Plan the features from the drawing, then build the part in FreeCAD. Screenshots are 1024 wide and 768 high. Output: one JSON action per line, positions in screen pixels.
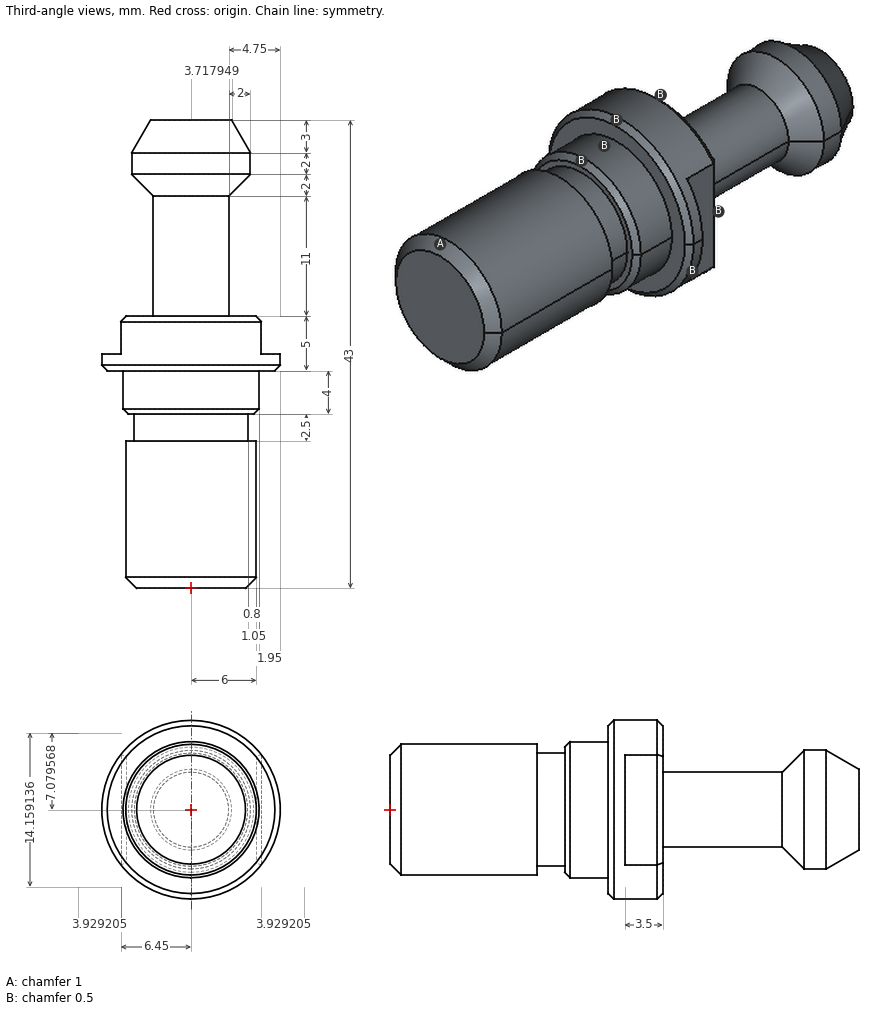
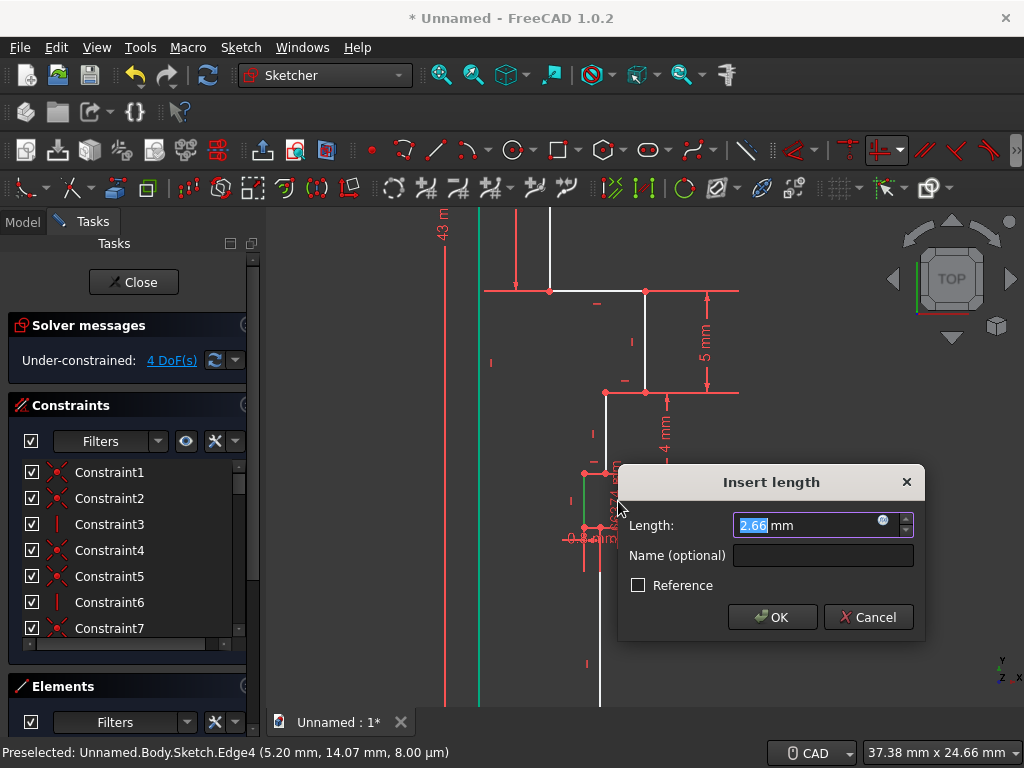
{"action": "type", "text": "2.5"}
{"action": "key", "text": "Return"}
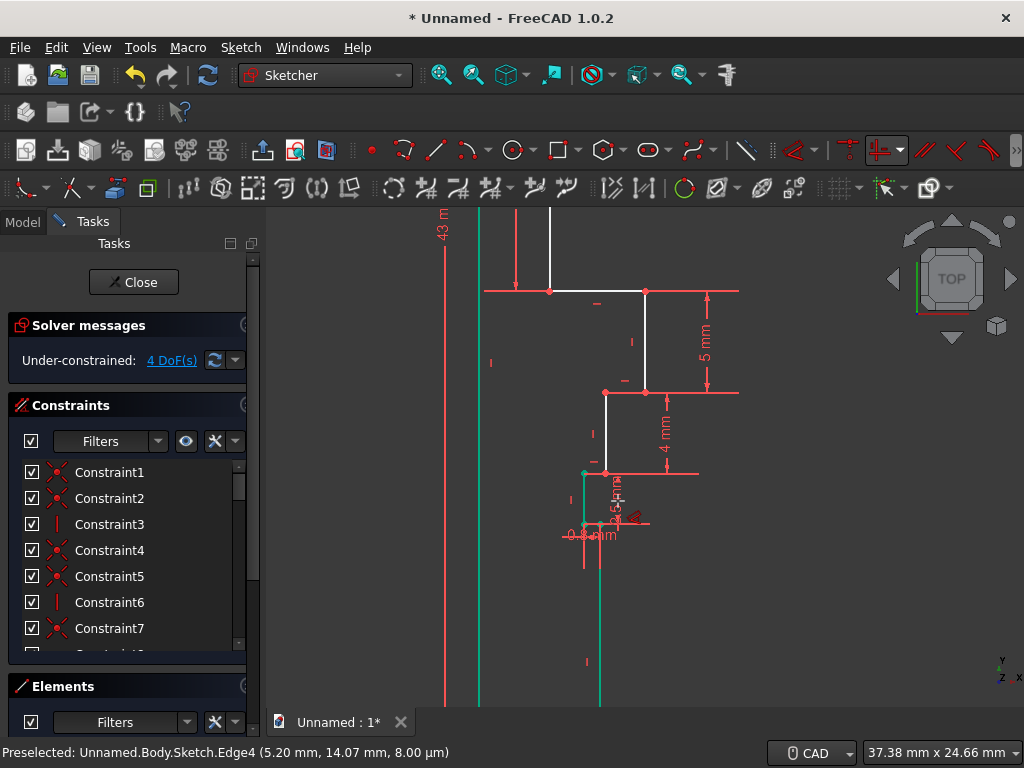
{"action": "scroll", "coordinate": [595, 474], "scroll_direction": "up", "scroll_amount": 4}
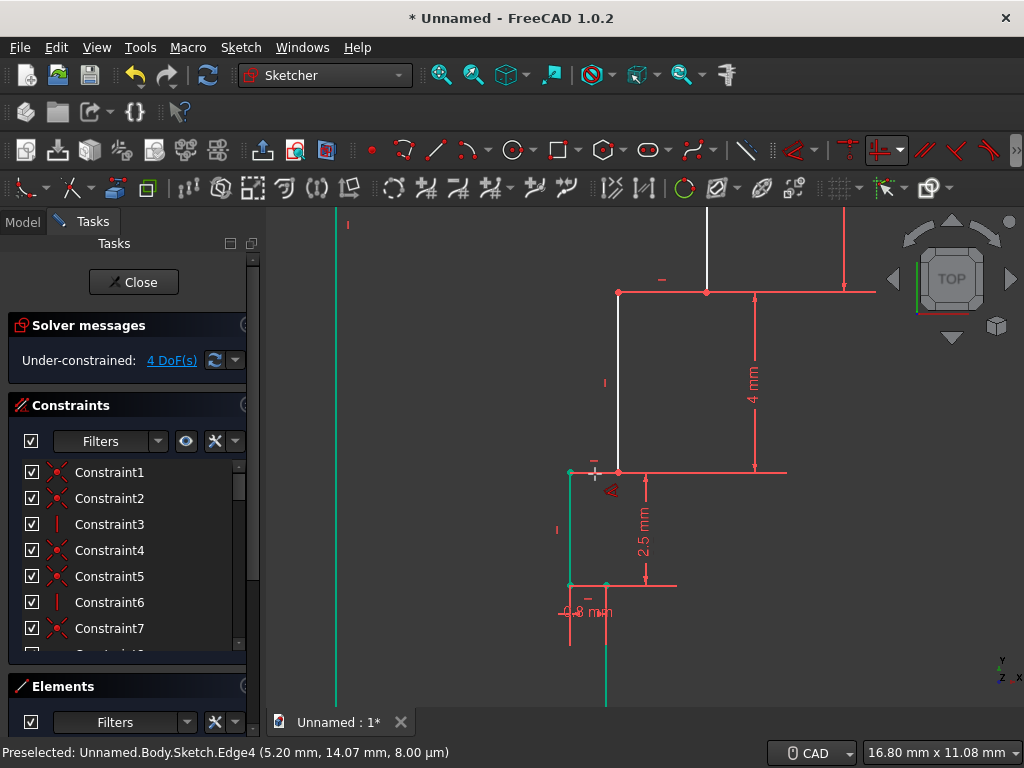
{"action": "left_click", "coordinate": [594, 473]}
{"action": "left_click", "coordinate": [594, 507]}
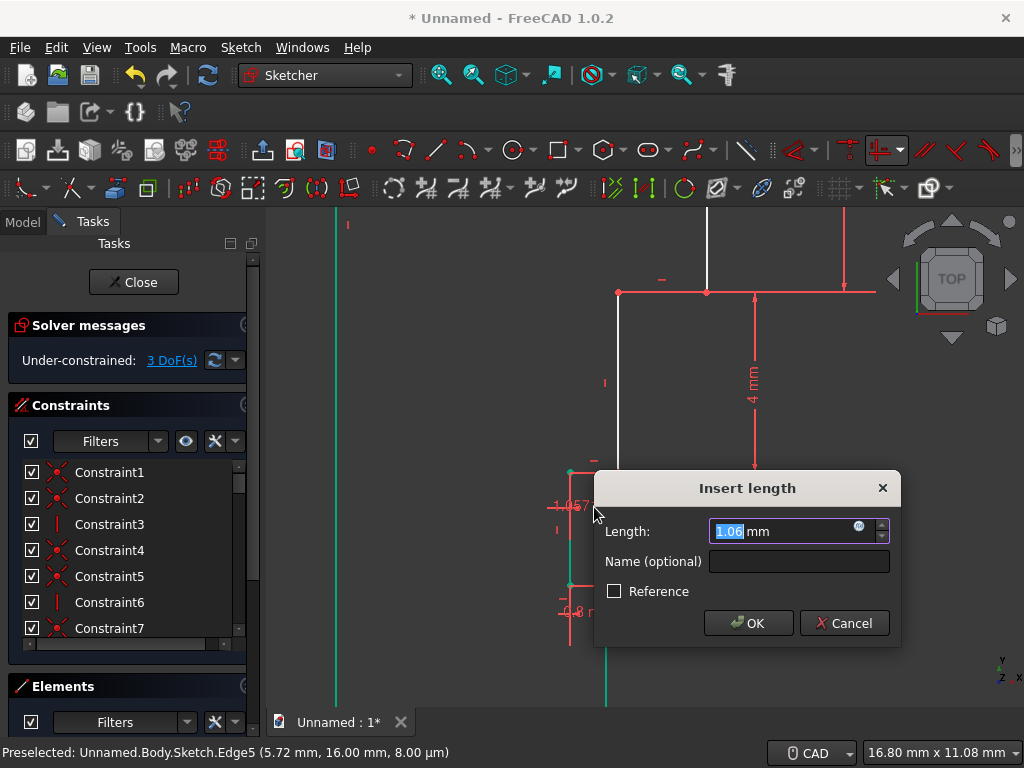
{"action": "type", "text": "1.05"}
{"action": "key", "text": "Return"}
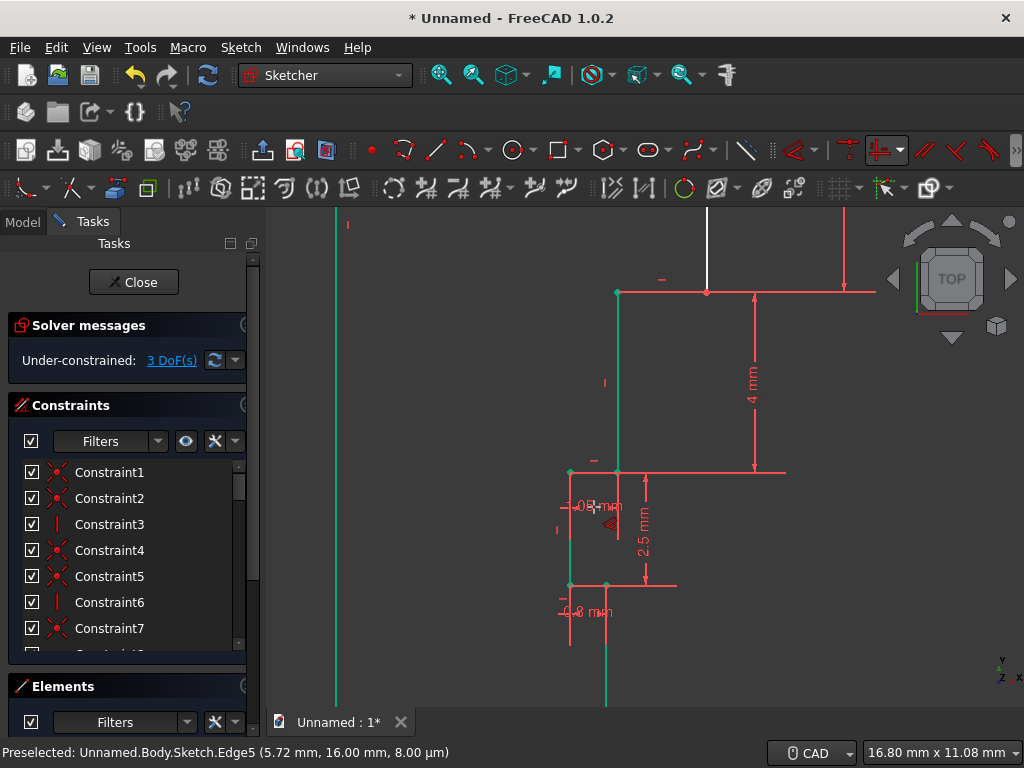
{"action": "left_click", "coordinate": [644, 292]}
{"action": "left_click", "coordinate": [662, 326]}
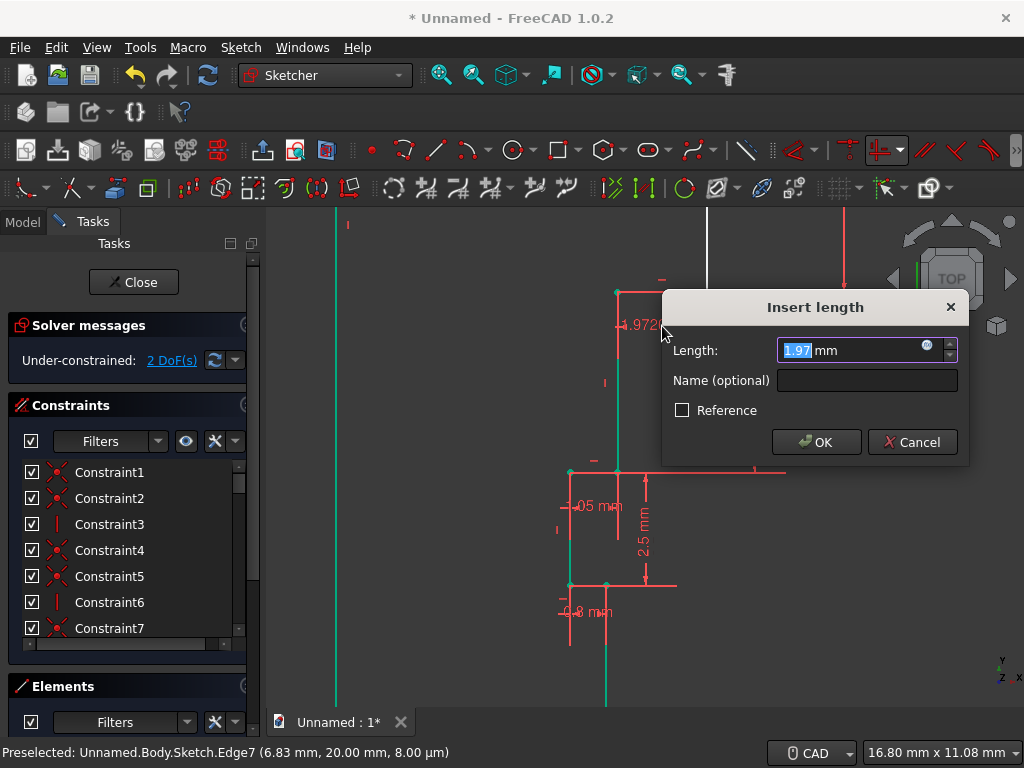
{"action": "type", "text": "1.95"}
{"action": "key", "text": "Return"}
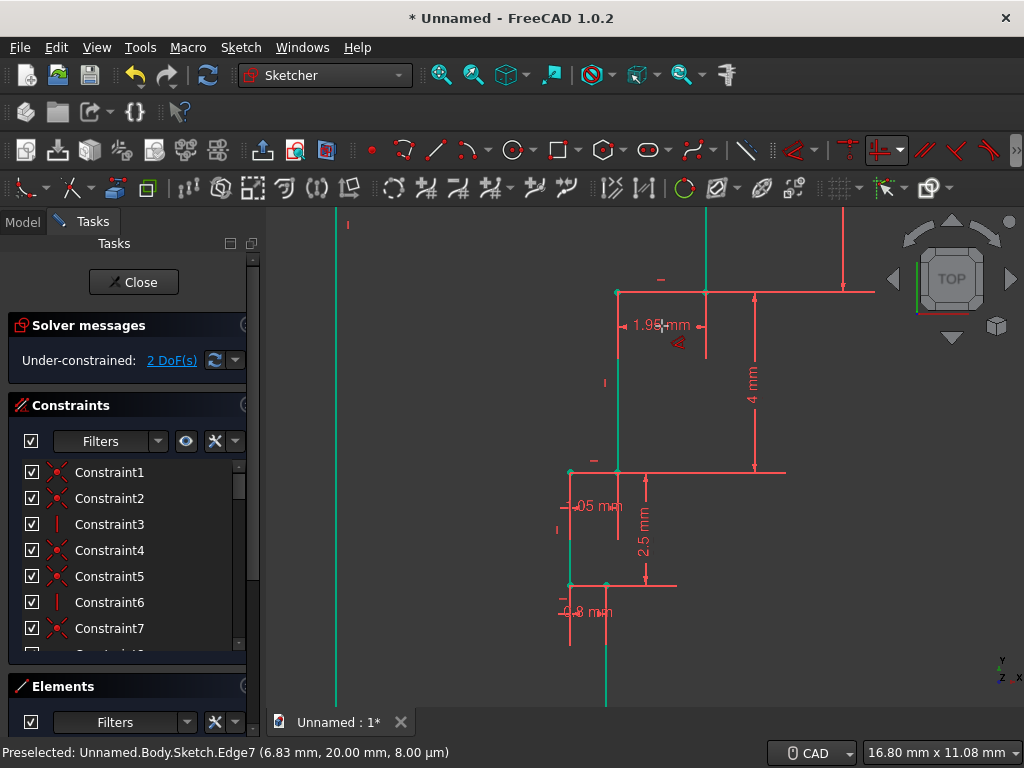
{"action": "scroll", "coordinate": [588, 503], "scroll_direction": "down", "scroll_amount": 9}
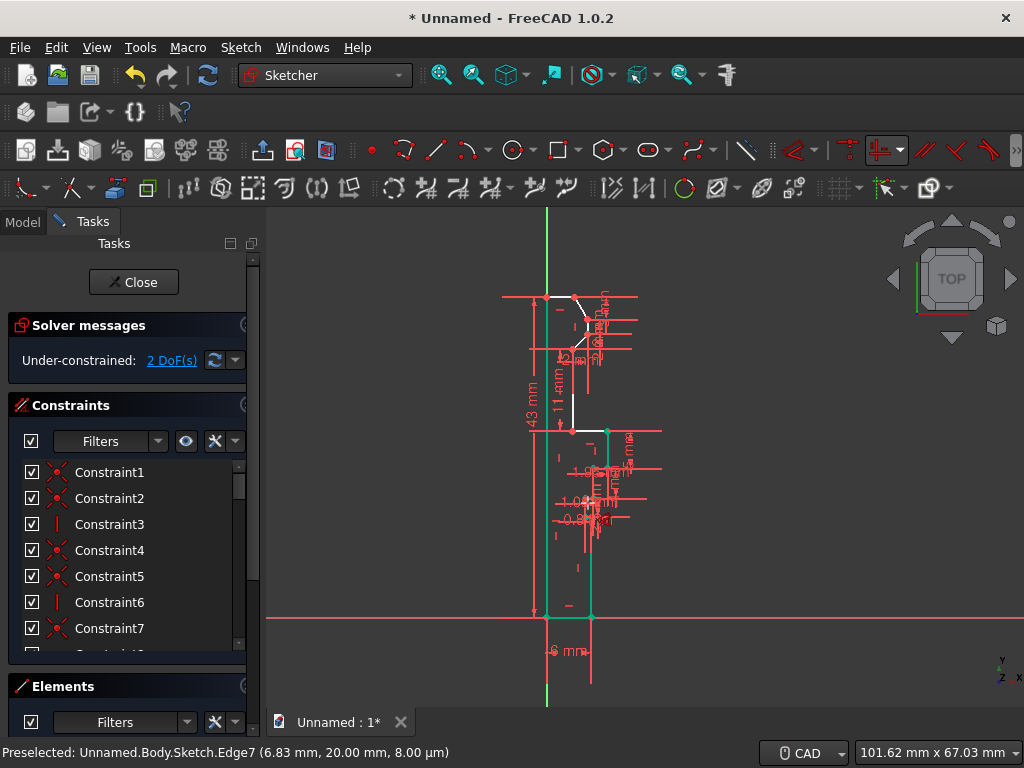
{"action": "scroll", "coordinate": [597, 431], "scroll_direction": "up", "scroll_amount": 2}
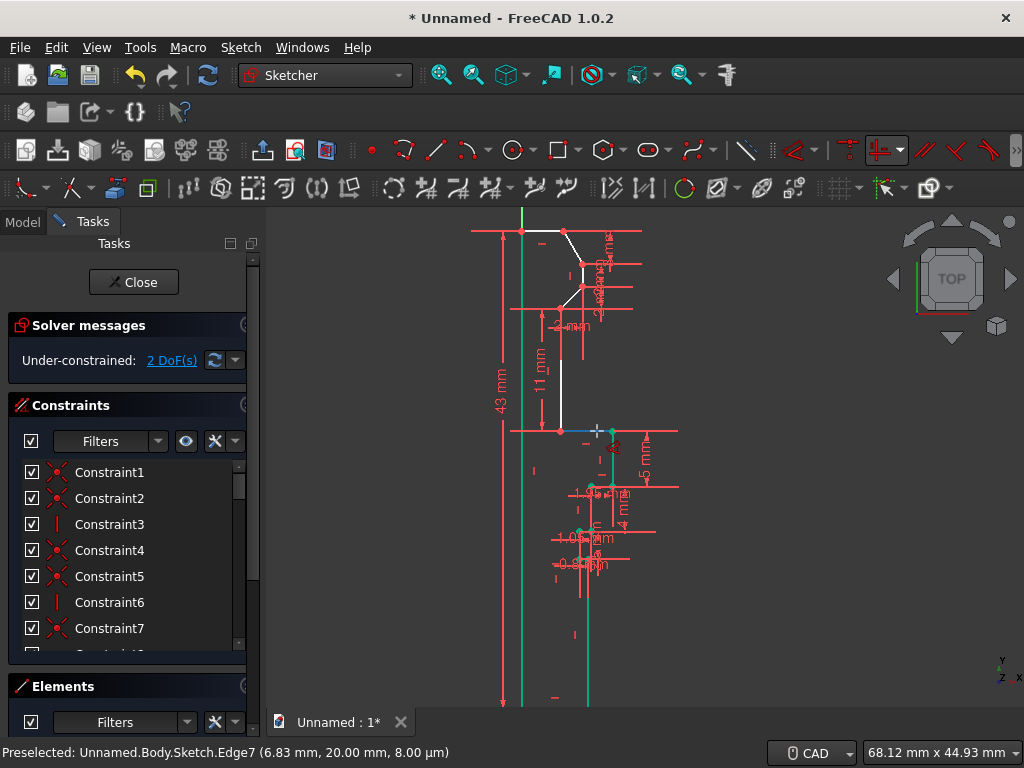
{"action": "left_click", "coordinate": [597, 431]}
{"action": "left_click", "coordinate": [587, 397]}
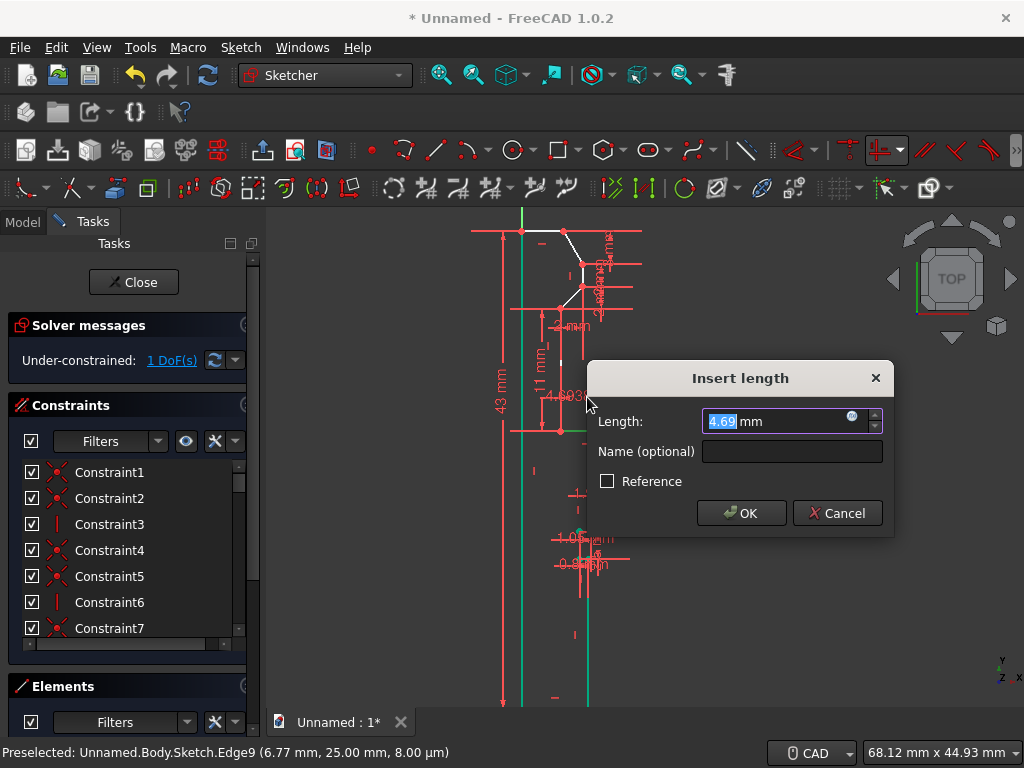
{"action": "type", "text": "4.75"}
{"action": "key", "text": "Return"}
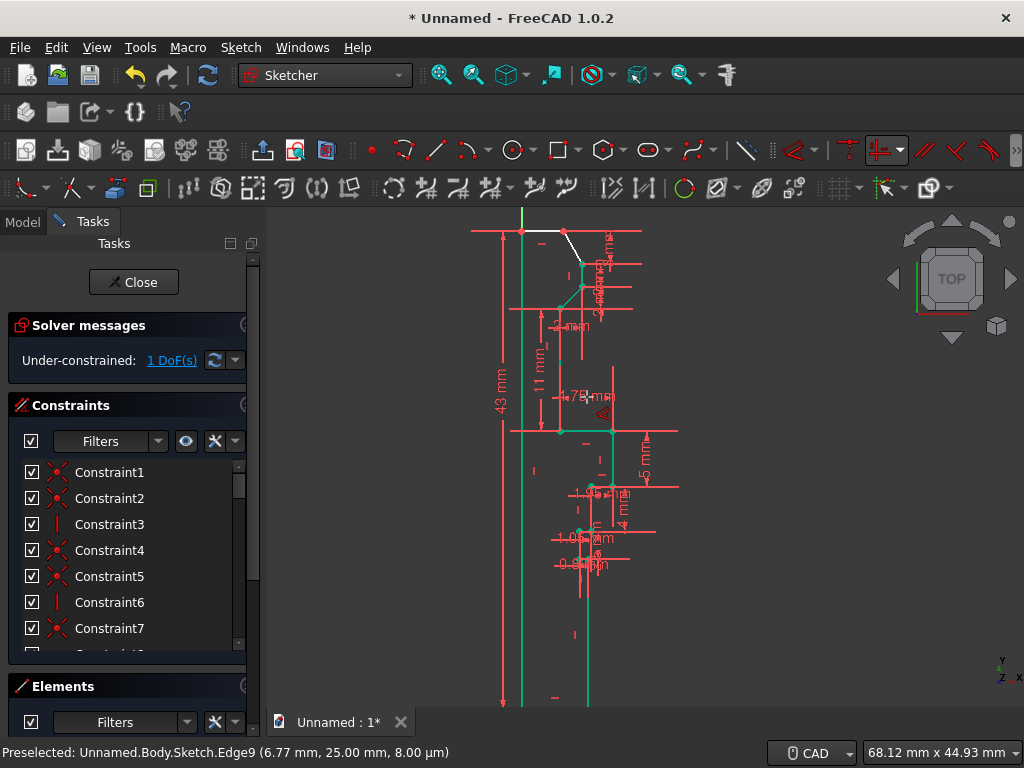
{"action": "scroll", "coordinate": [595, 430], "scroll_direction": "down", "scroll_amount": 2}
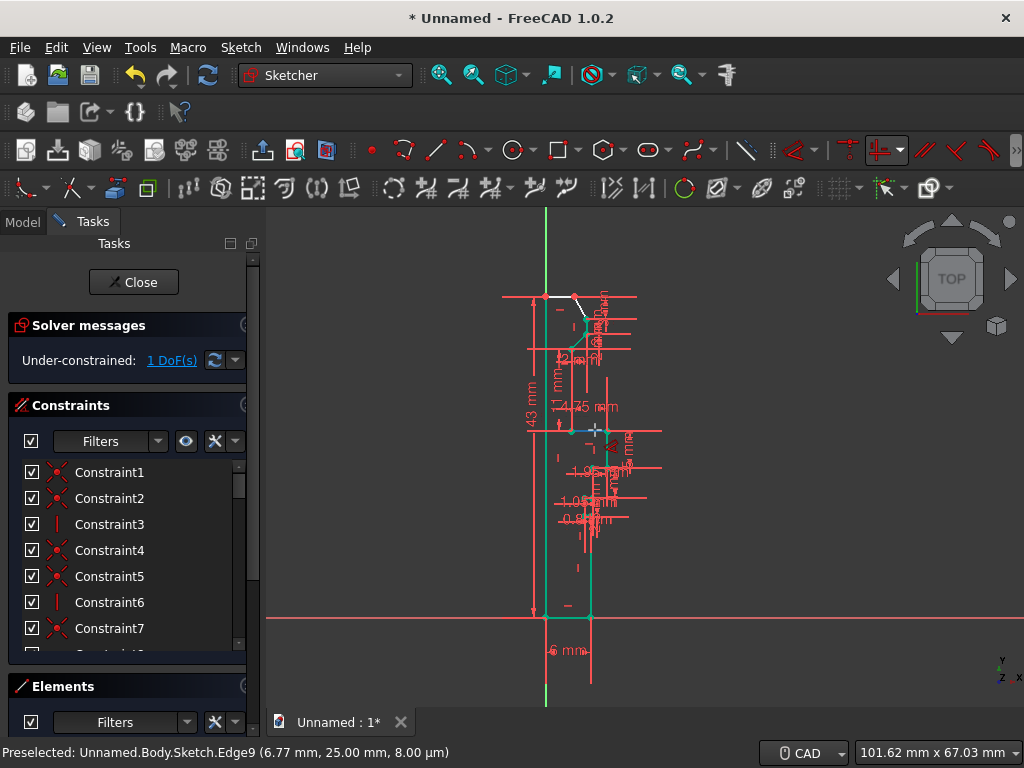
{"action": "scroll", "coordinate": [566, 297], "scroll_direction": "up", "scroll_amount": 3}